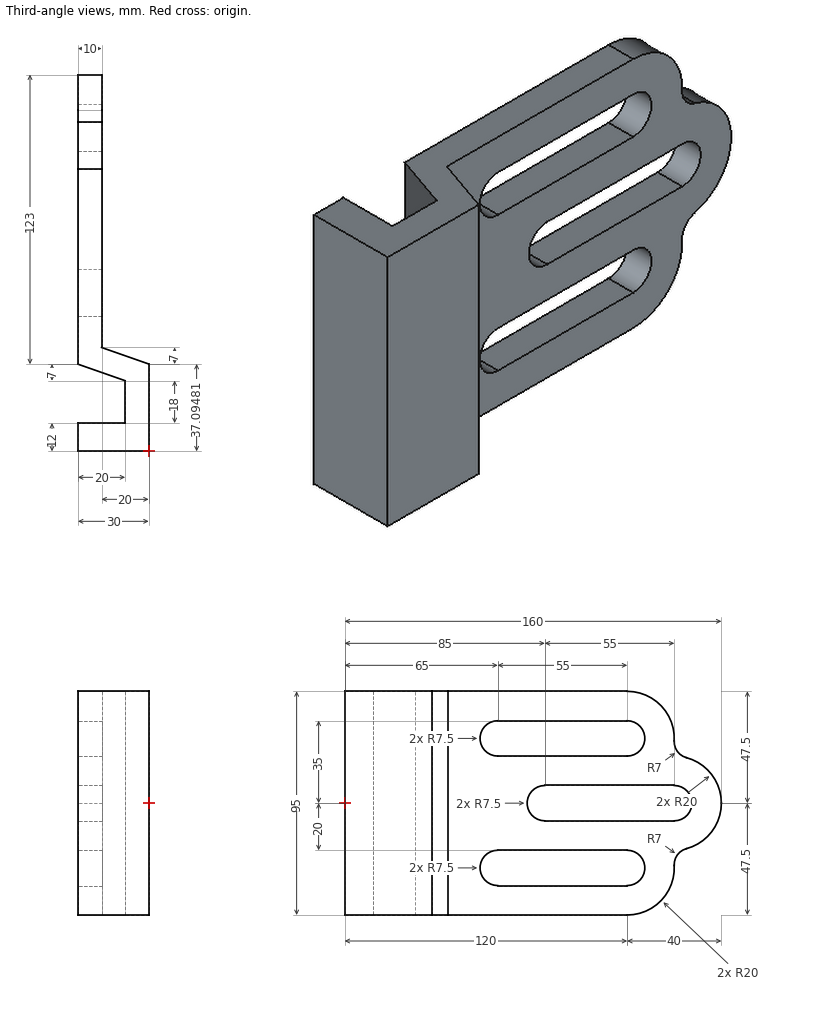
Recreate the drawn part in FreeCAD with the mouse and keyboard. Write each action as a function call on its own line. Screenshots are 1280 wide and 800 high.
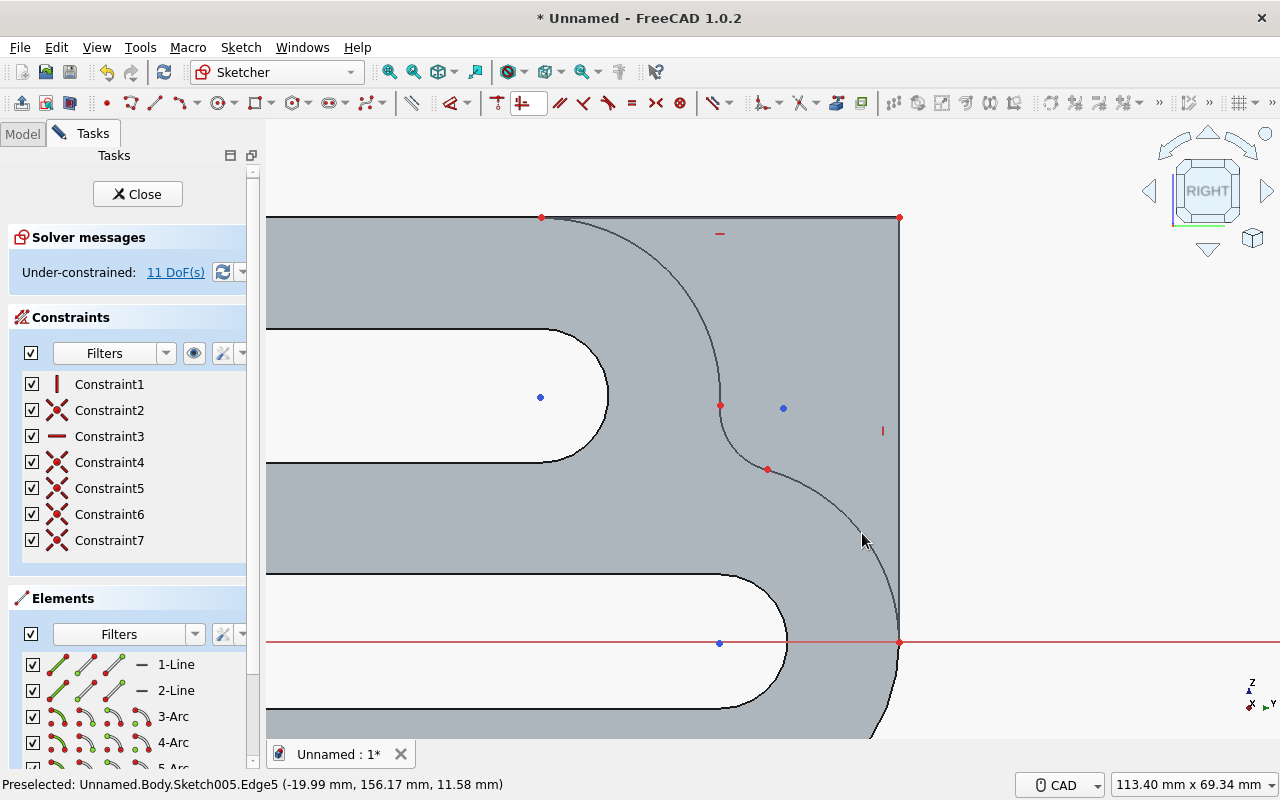
click(899, 515)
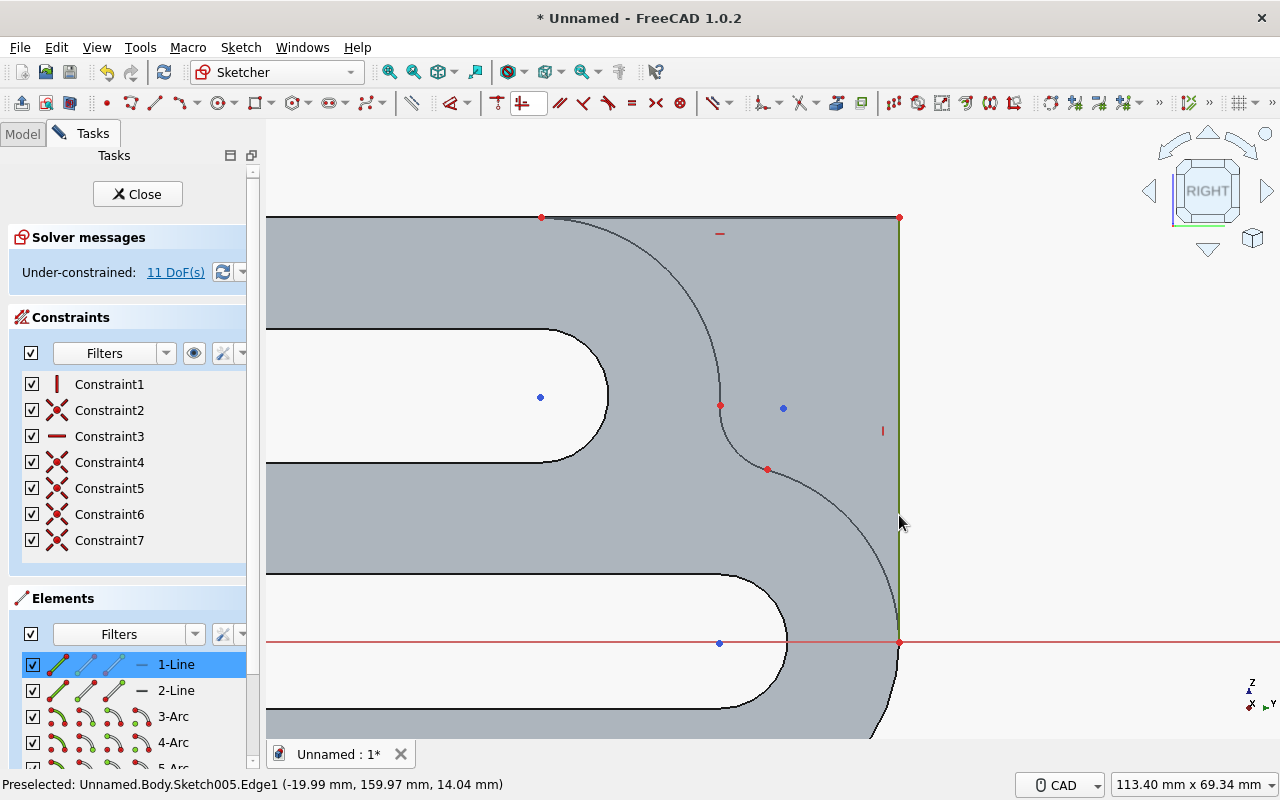
click(885, 575)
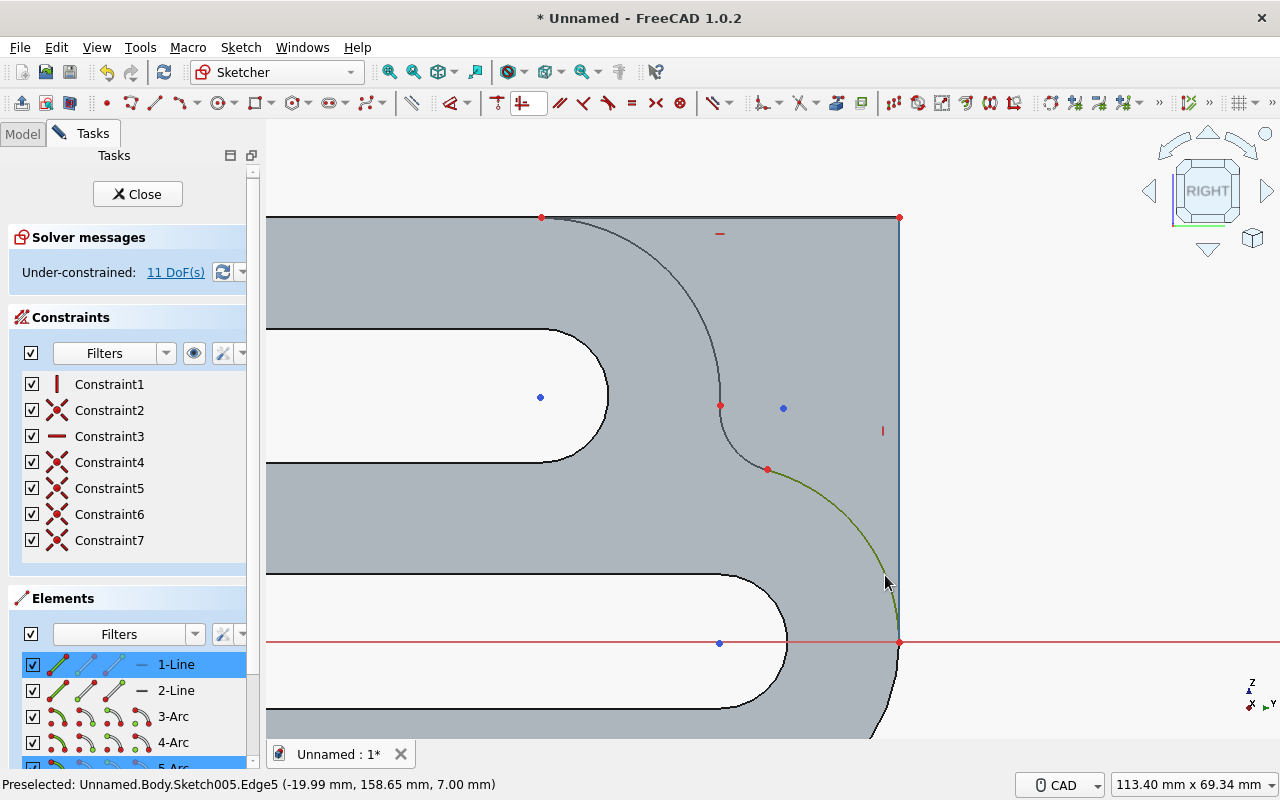
click(608, 104)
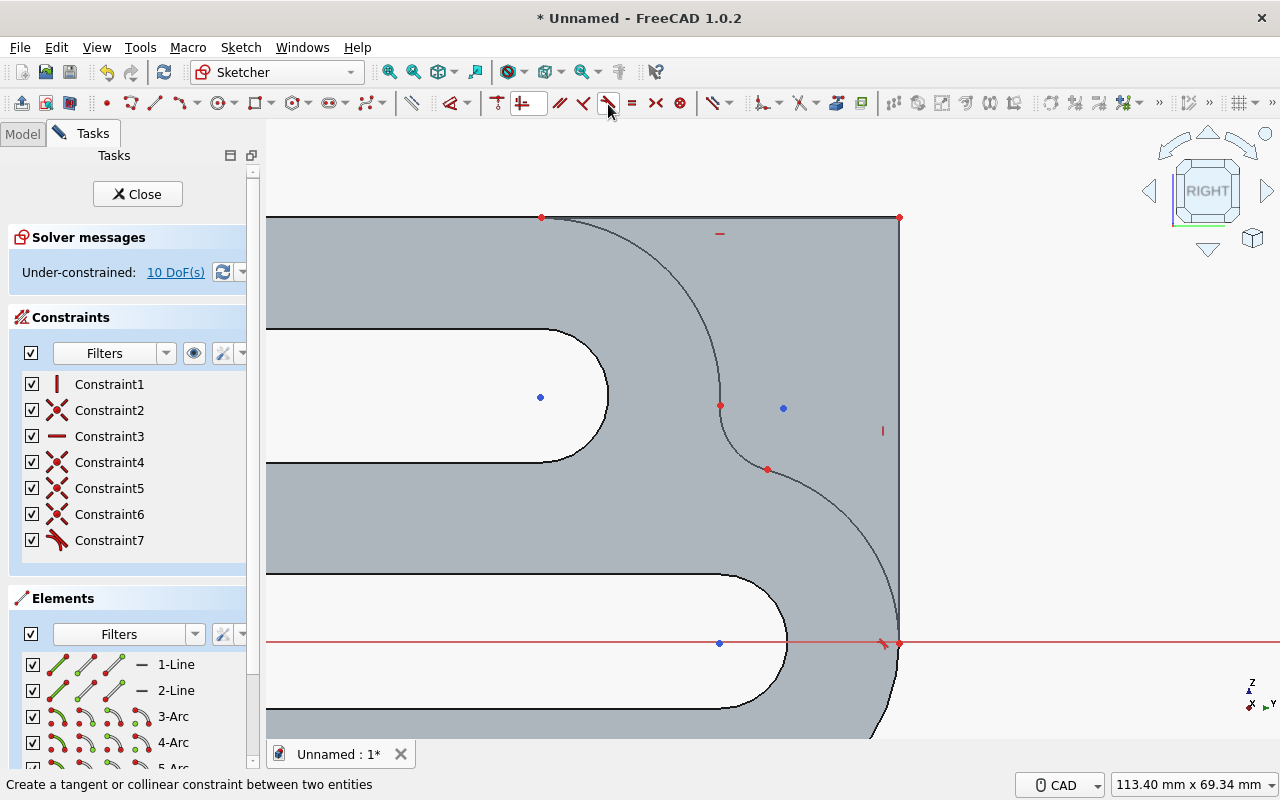
click(792, 218)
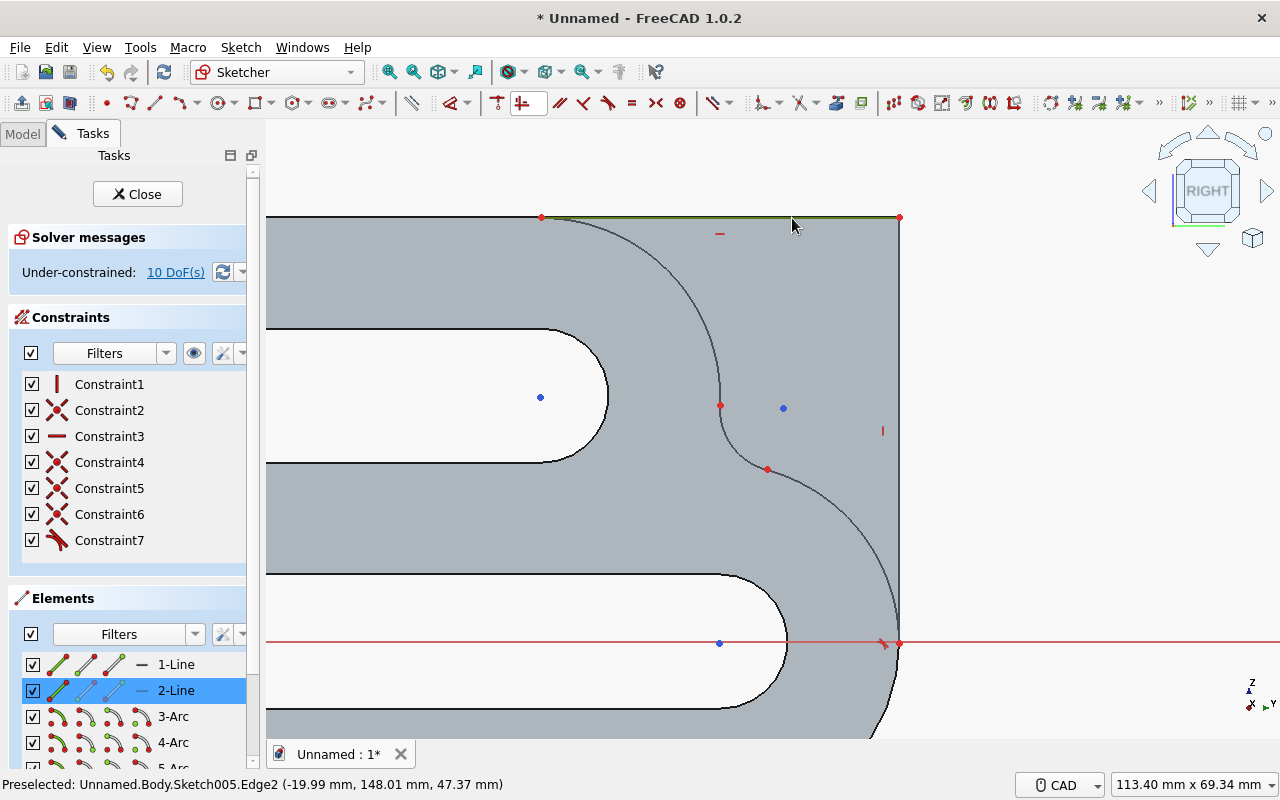
click(703, 322)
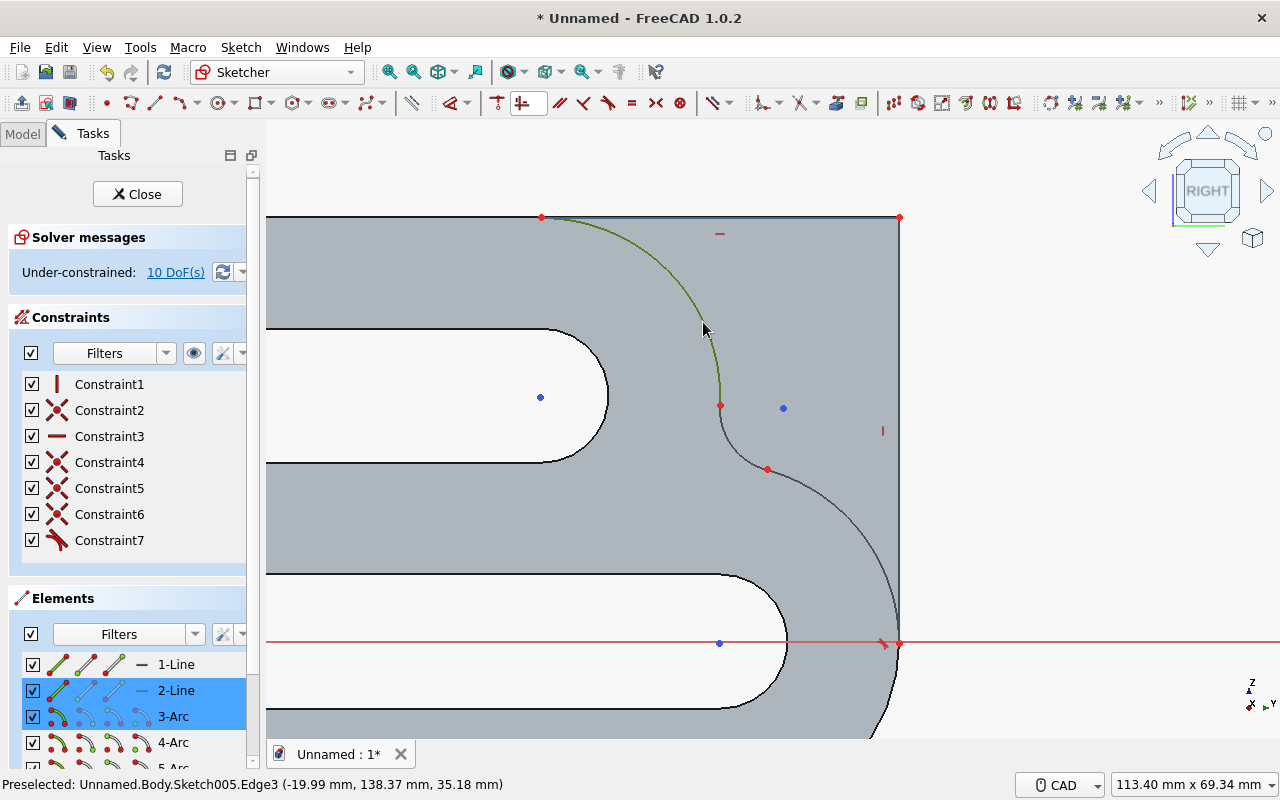
key(t)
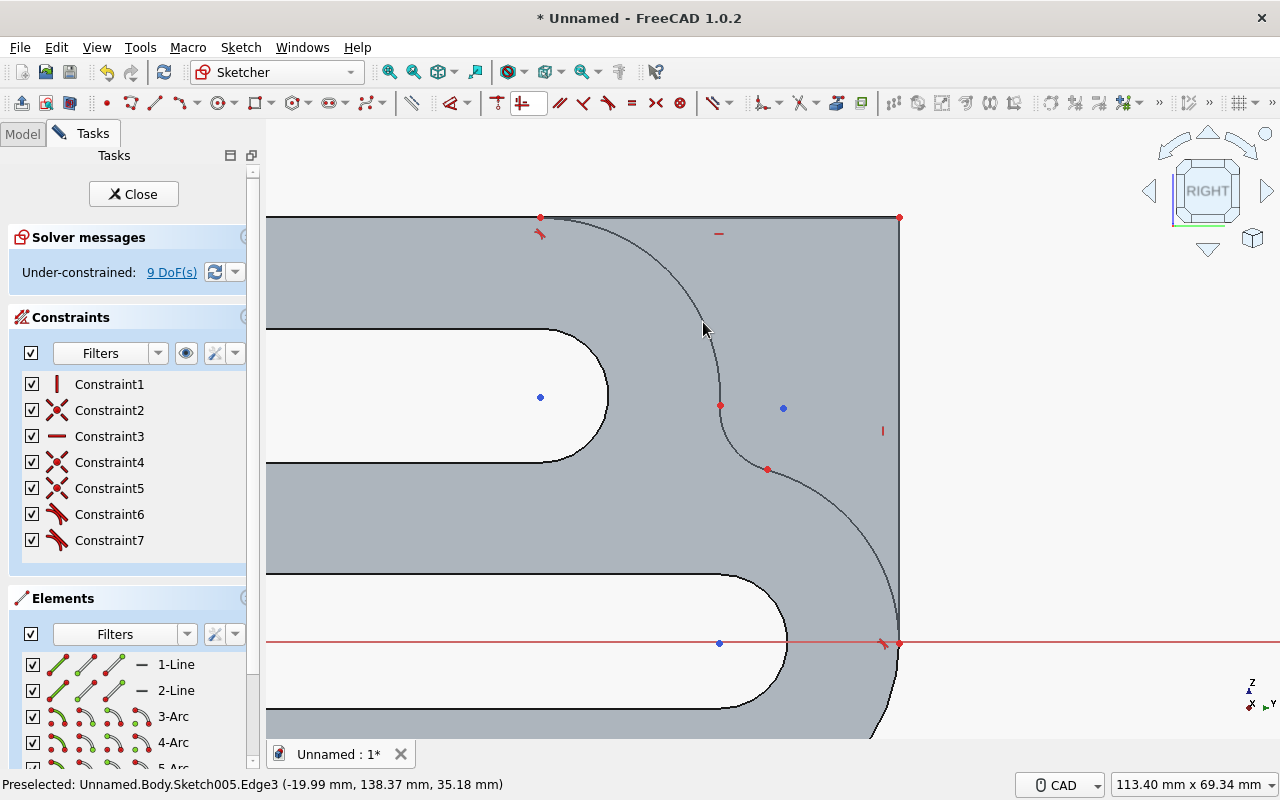
click(703, 321)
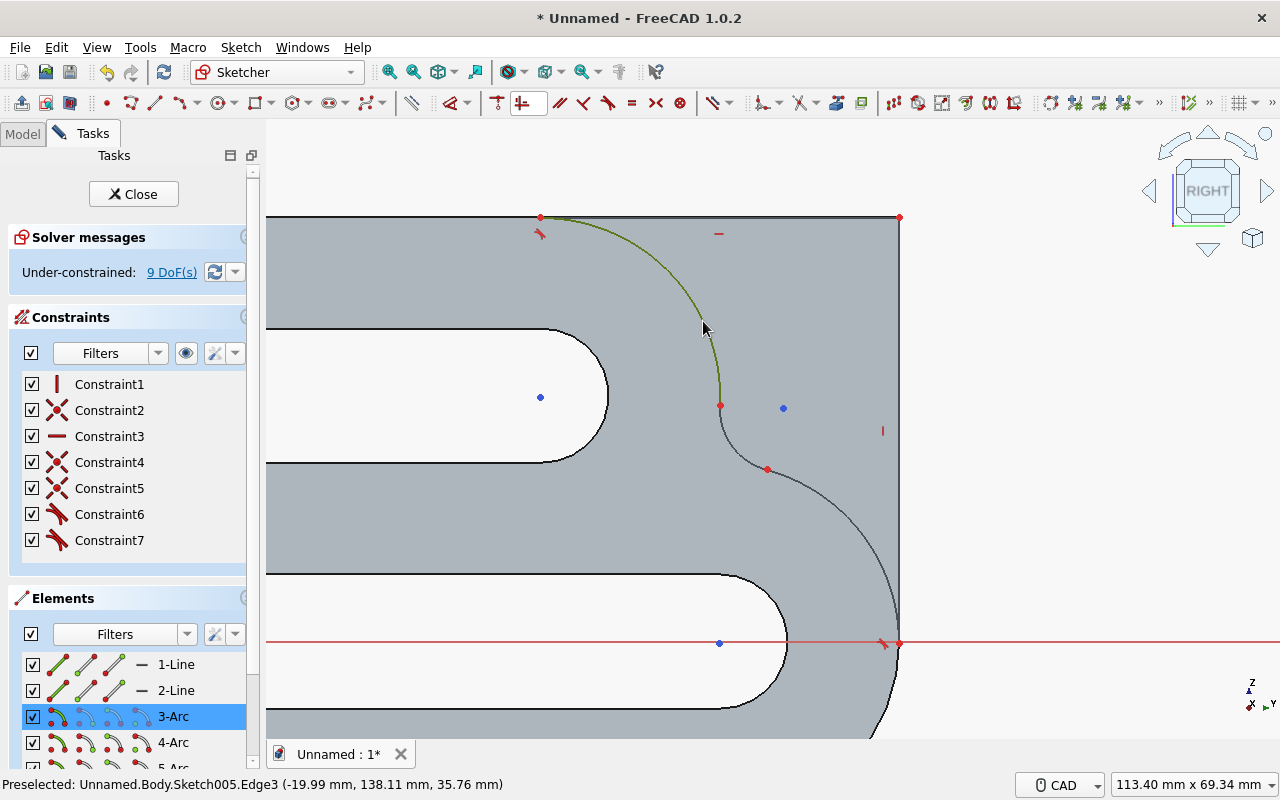
click(724, 431)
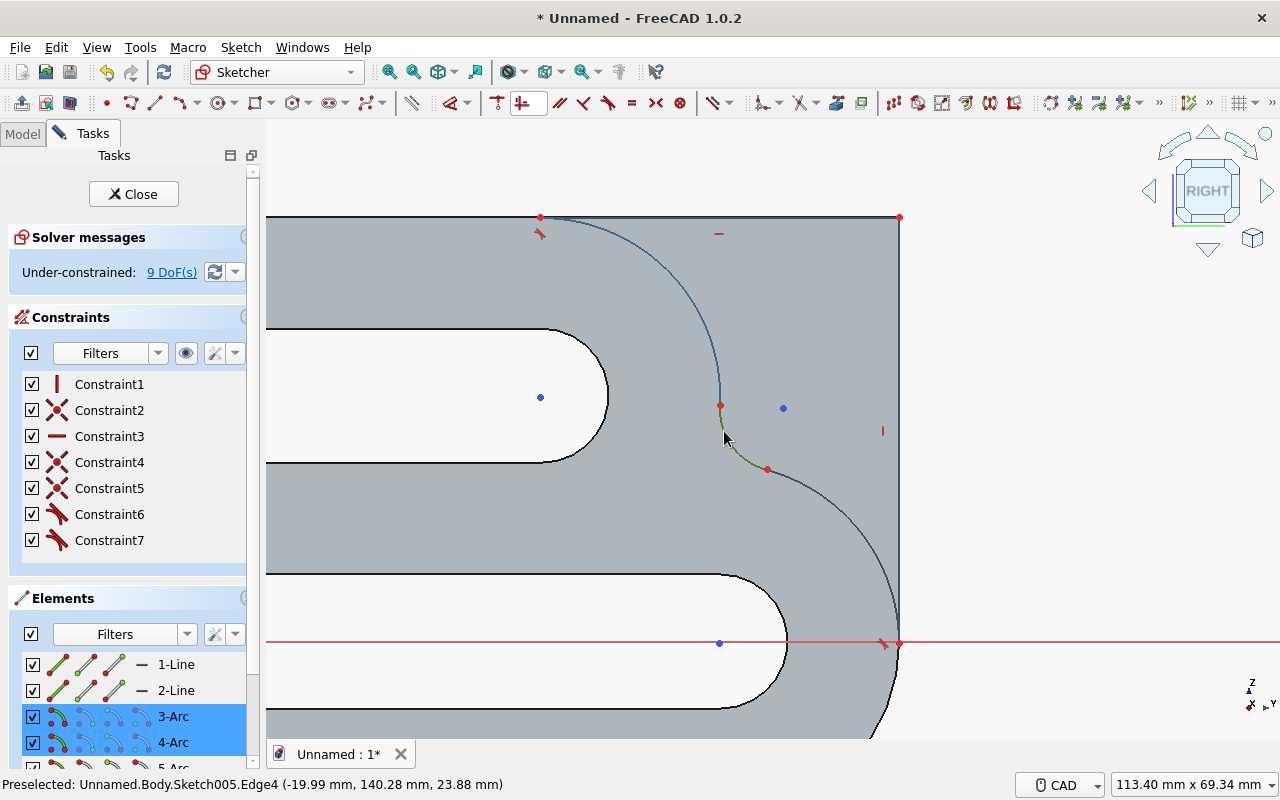
click(608, 104)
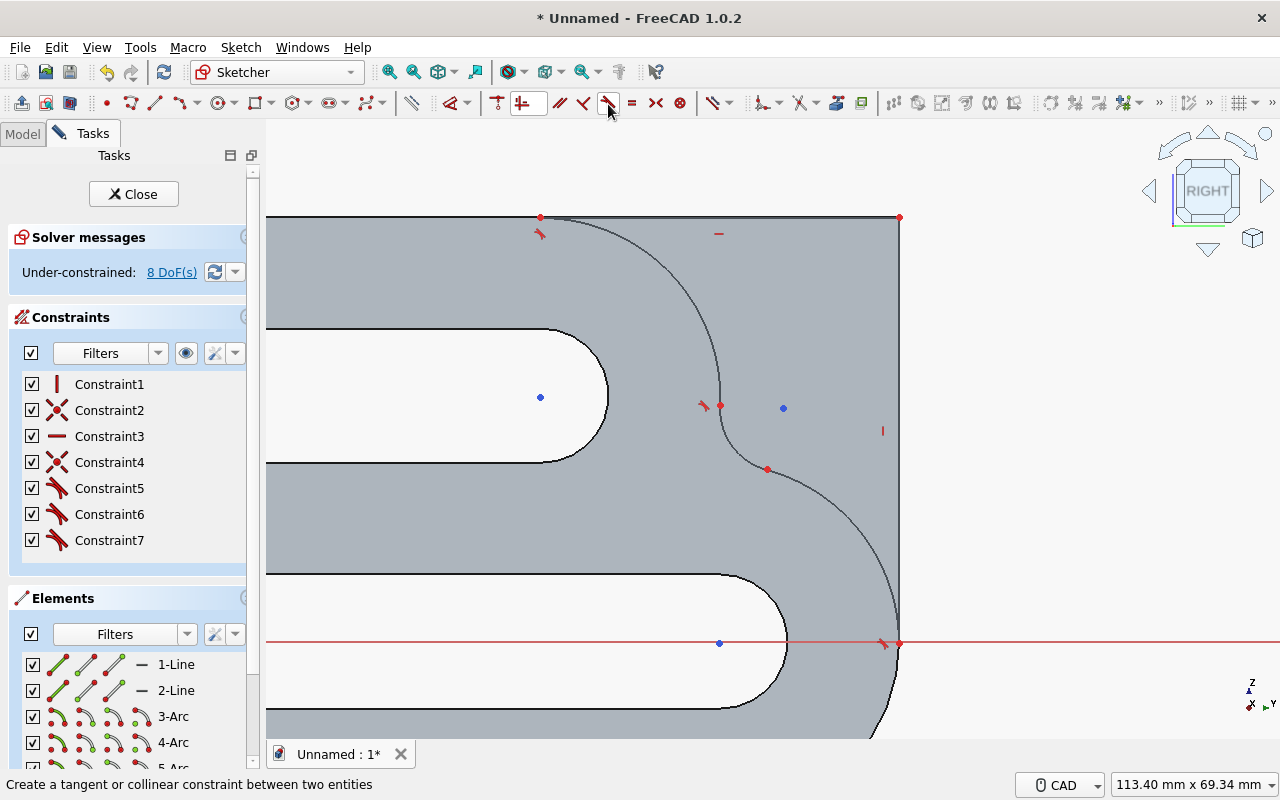
click(724, 431)